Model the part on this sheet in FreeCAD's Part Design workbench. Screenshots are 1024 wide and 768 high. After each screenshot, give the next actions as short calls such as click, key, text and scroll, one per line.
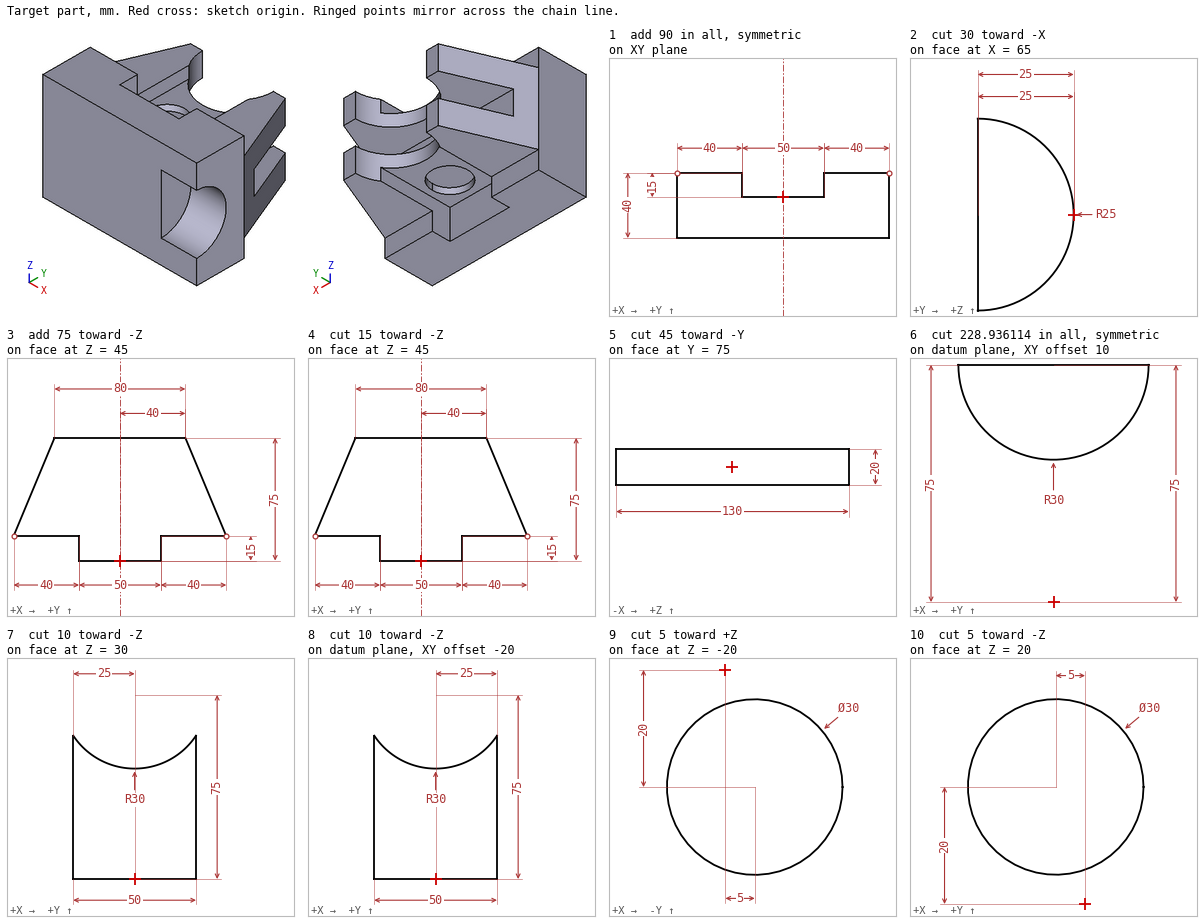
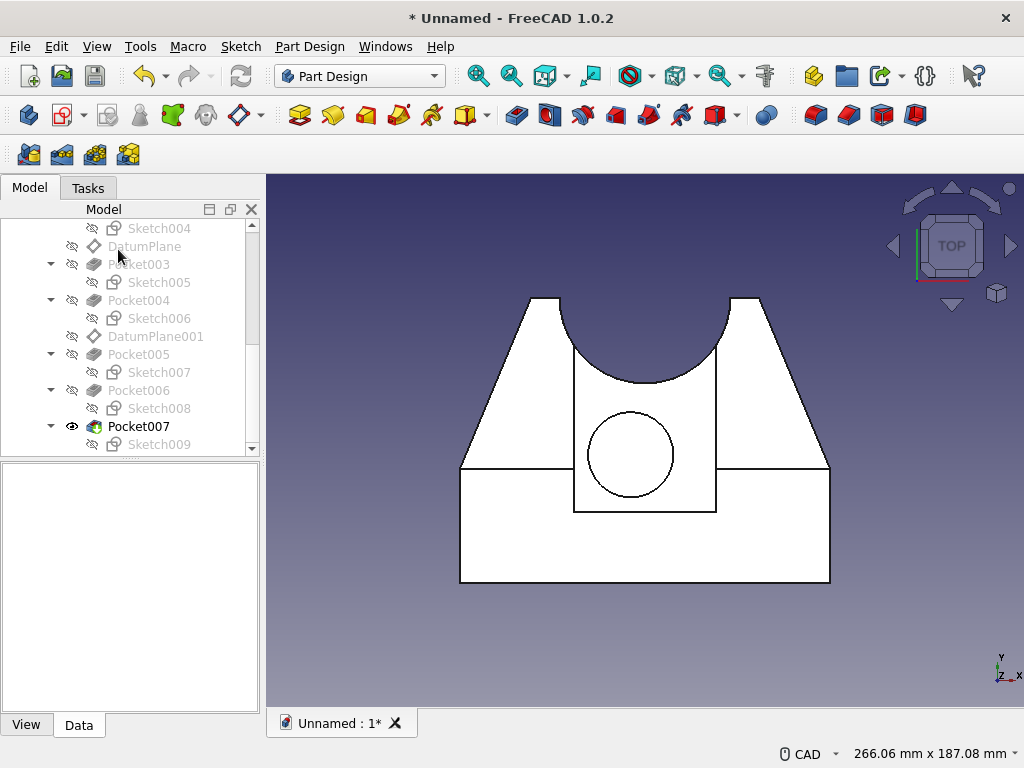
key(0)